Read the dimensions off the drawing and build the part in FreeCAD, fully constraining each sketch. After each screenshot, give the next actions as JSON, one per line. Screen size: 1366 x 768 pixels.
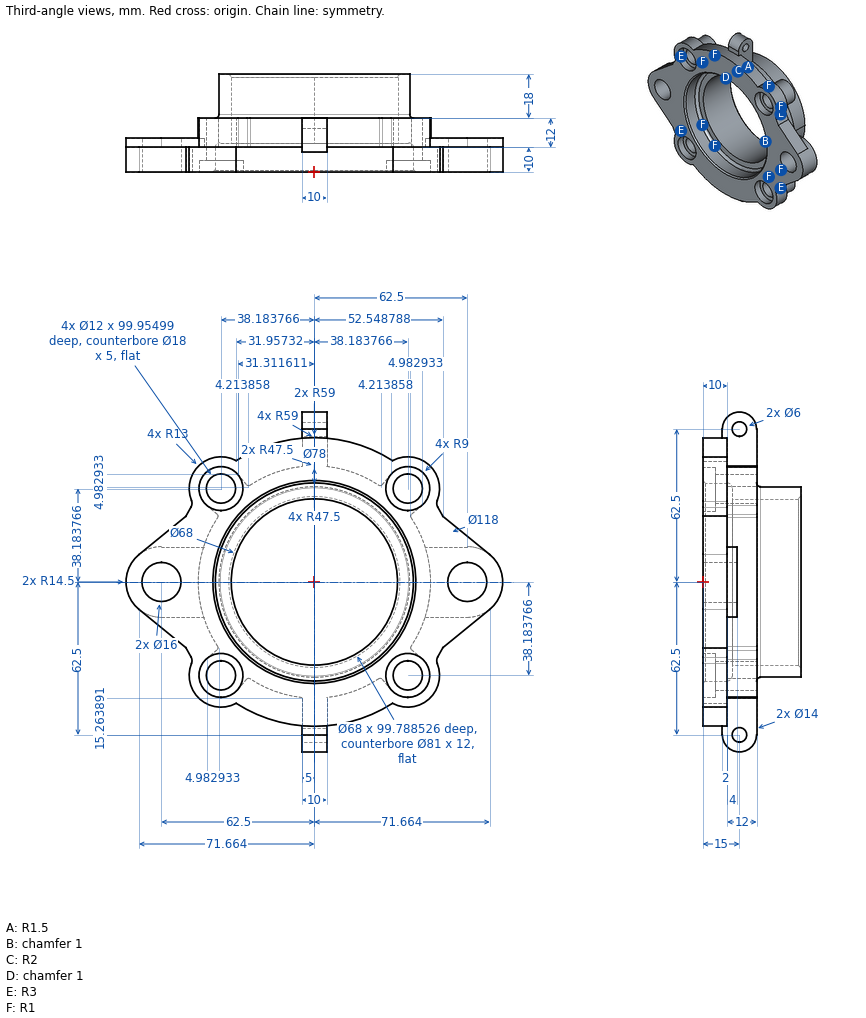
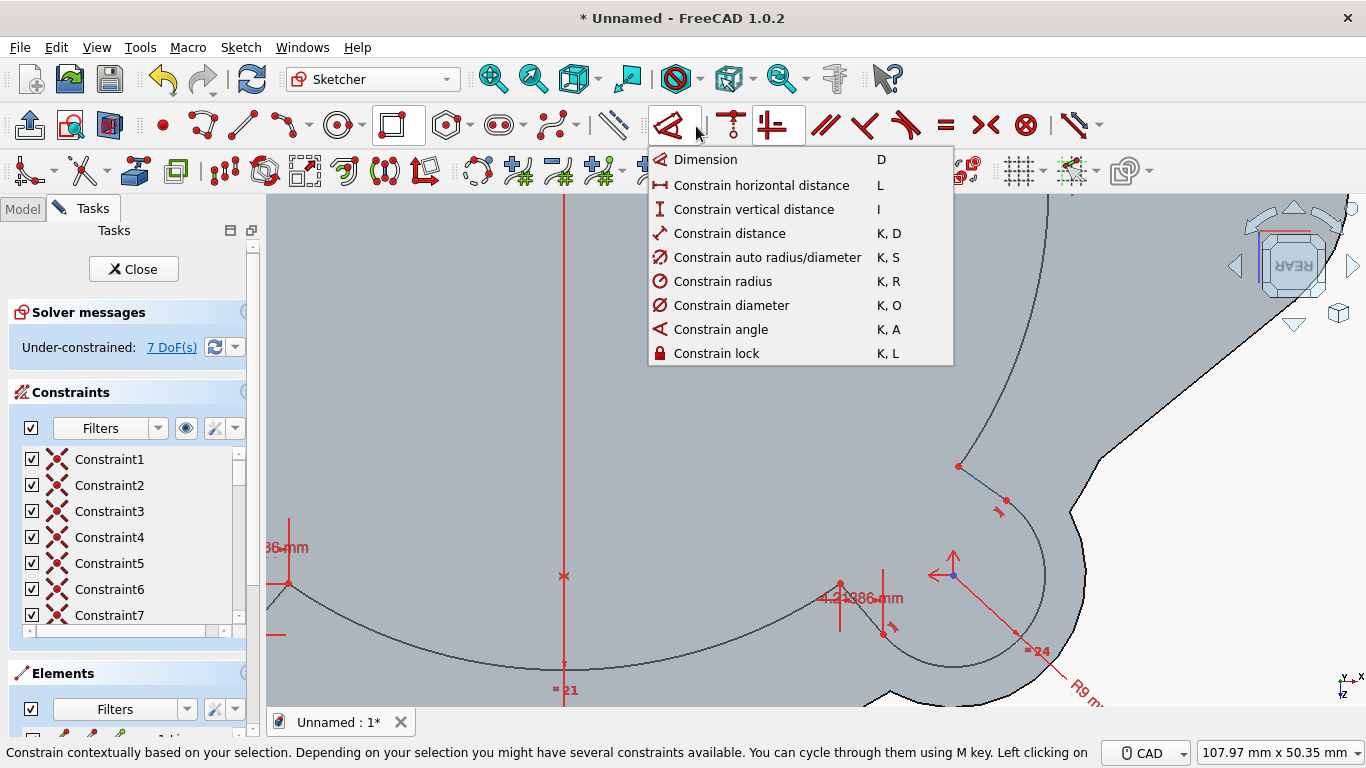
{"action": "left_click", "coordinate": [801, 185]}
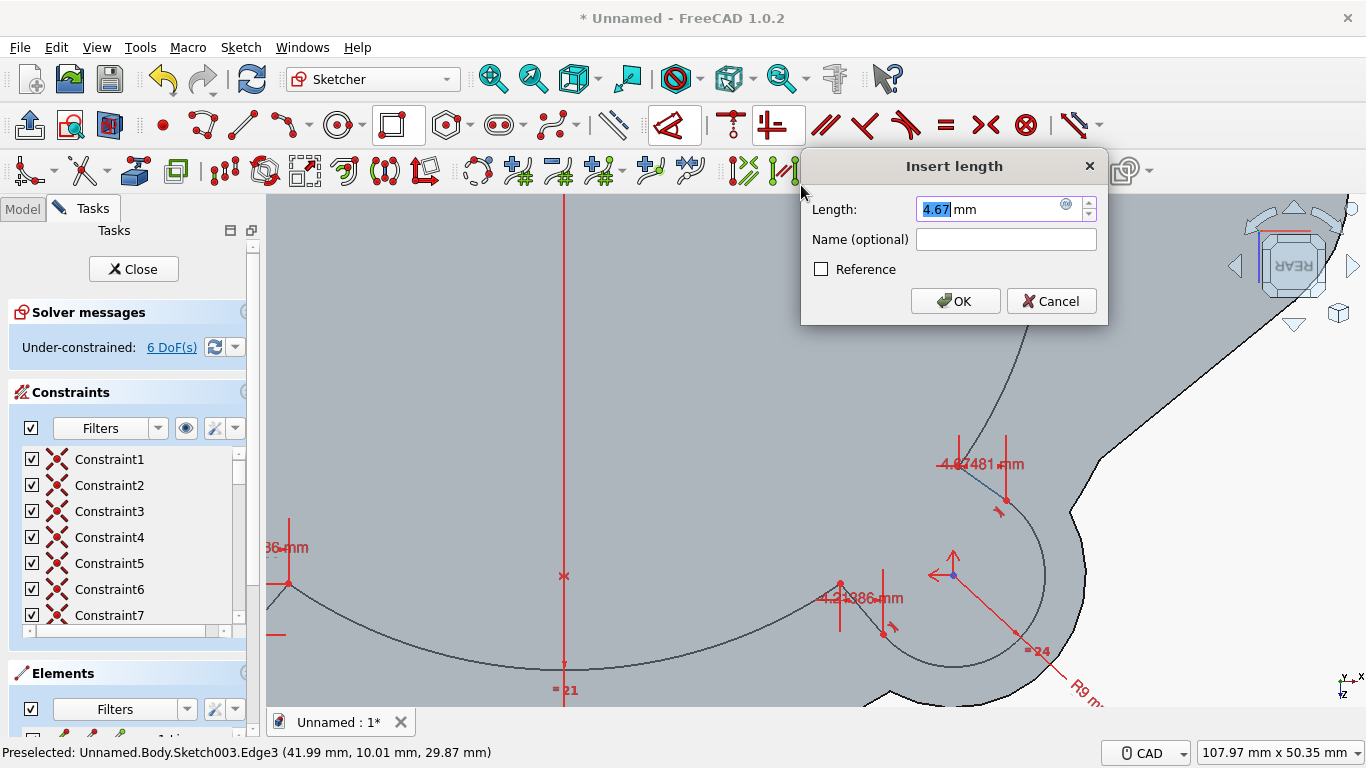
{"action": "type", "text": "4.982933"}
{"action": "key", "text": "Return"}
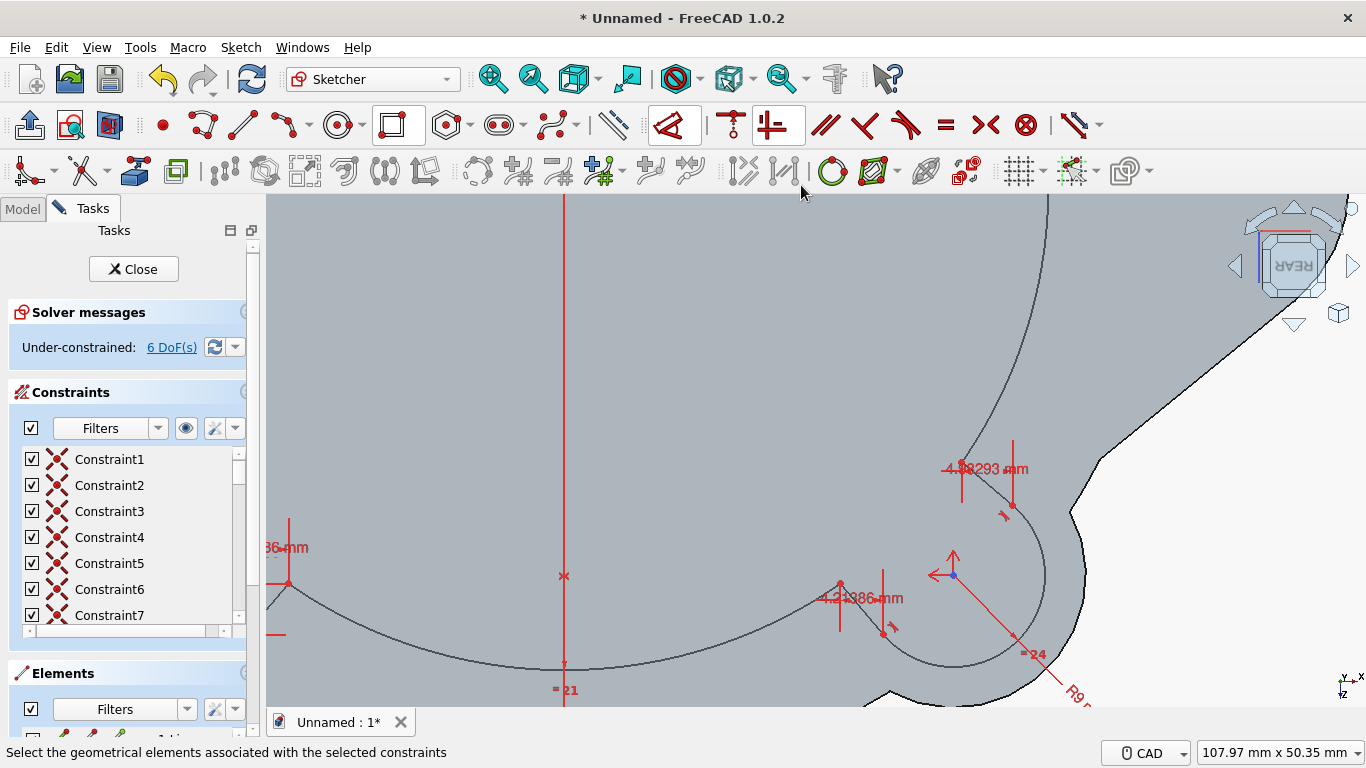
{"action": "scroll", "coordinate": [854, 604], "scroll_direction": "down", "scroll_amount": 5}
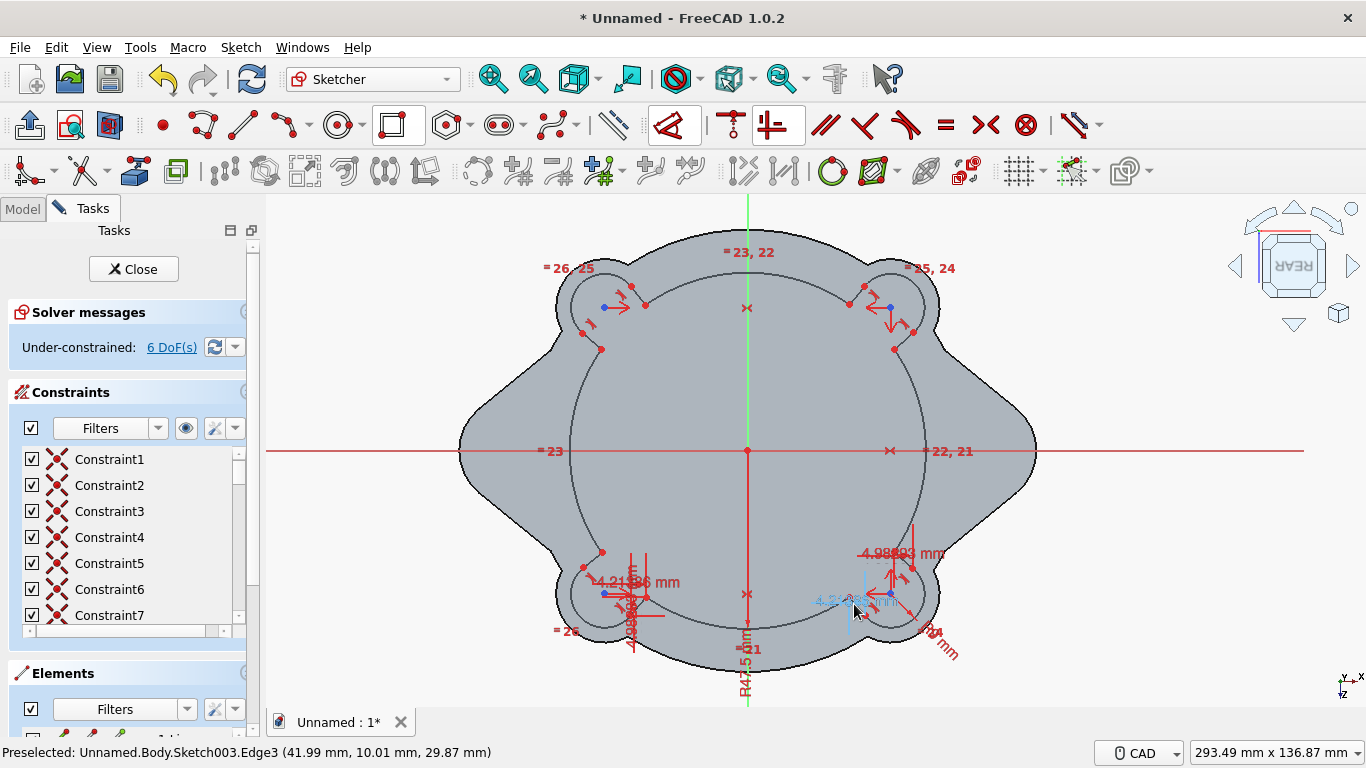
{"action": "scroll", "coordinate": [900, 345], "scroll_direction": "up", "scroll_amount": 4}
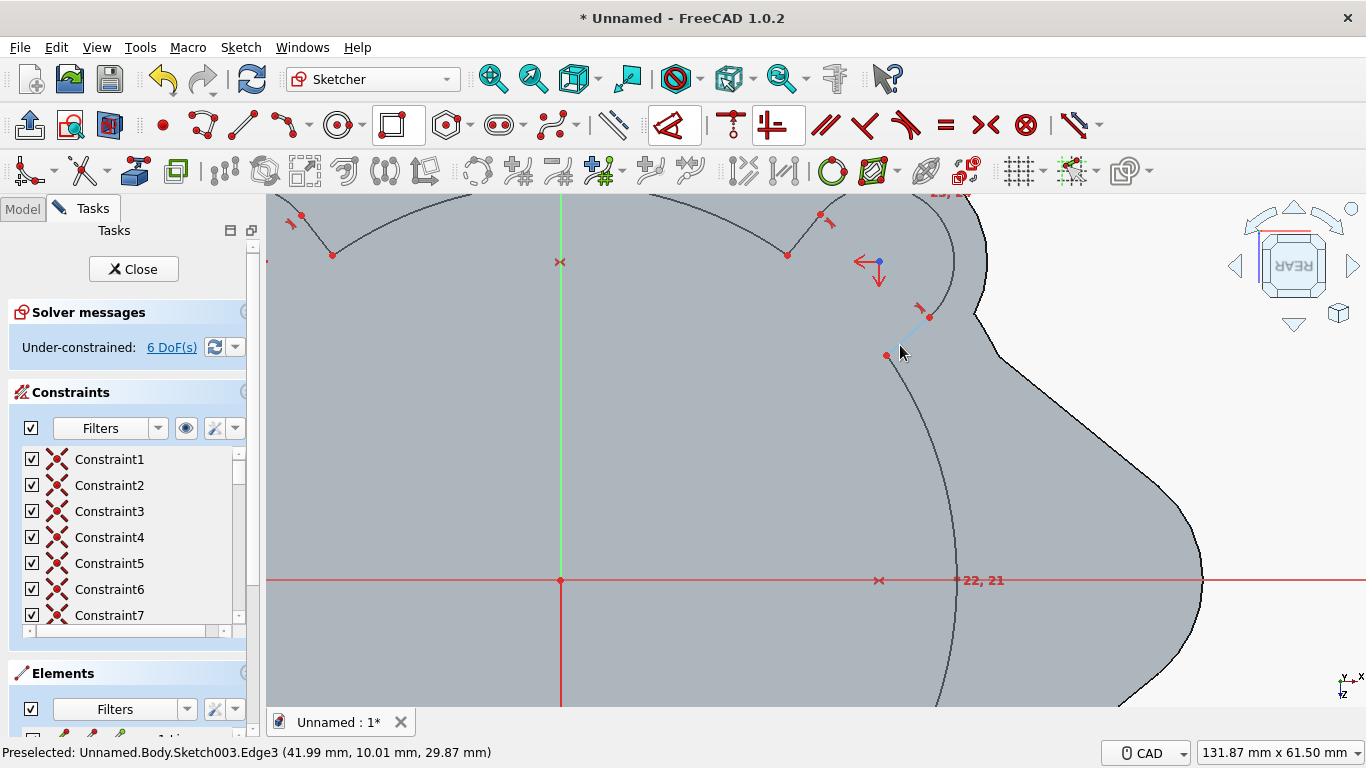
{"action": "left_click", "coordinate": [900, 344]}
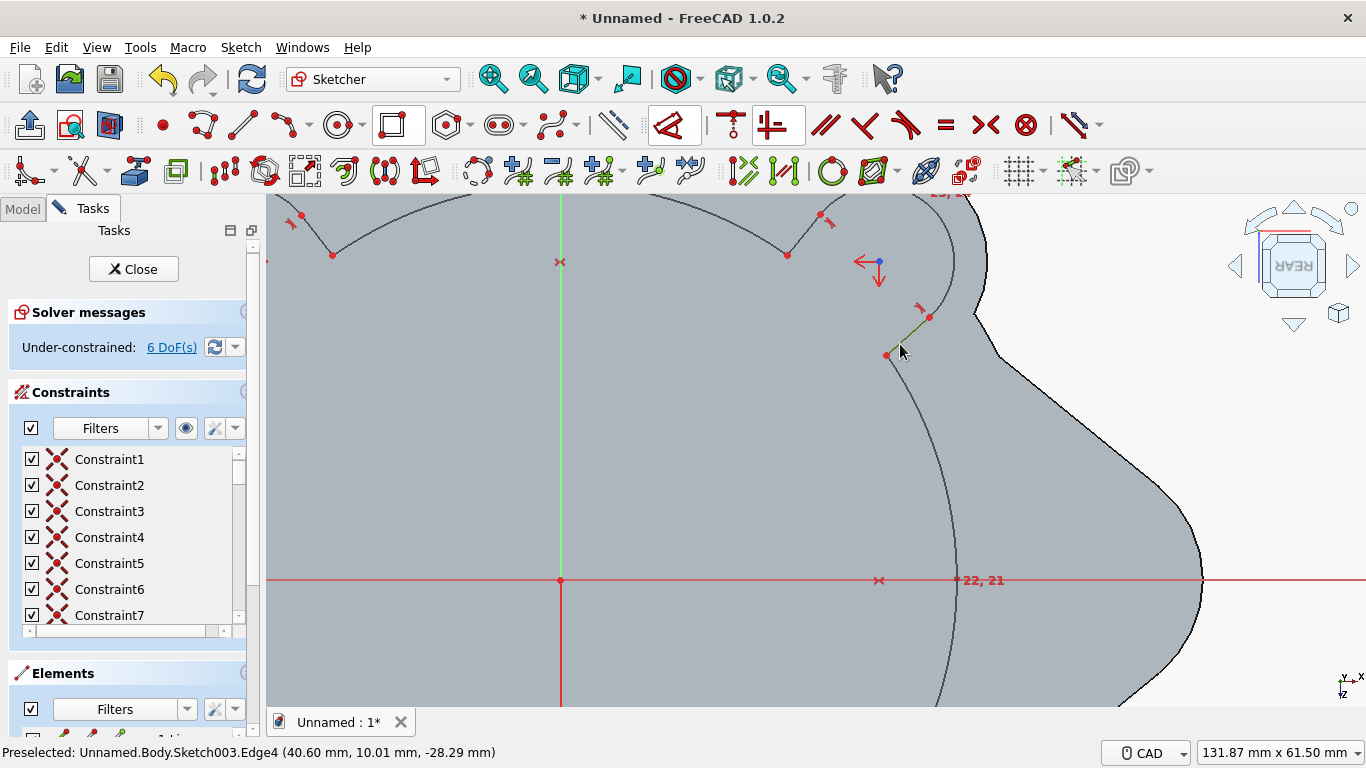
{"action": "left_click", "coordinate": [696, 126]}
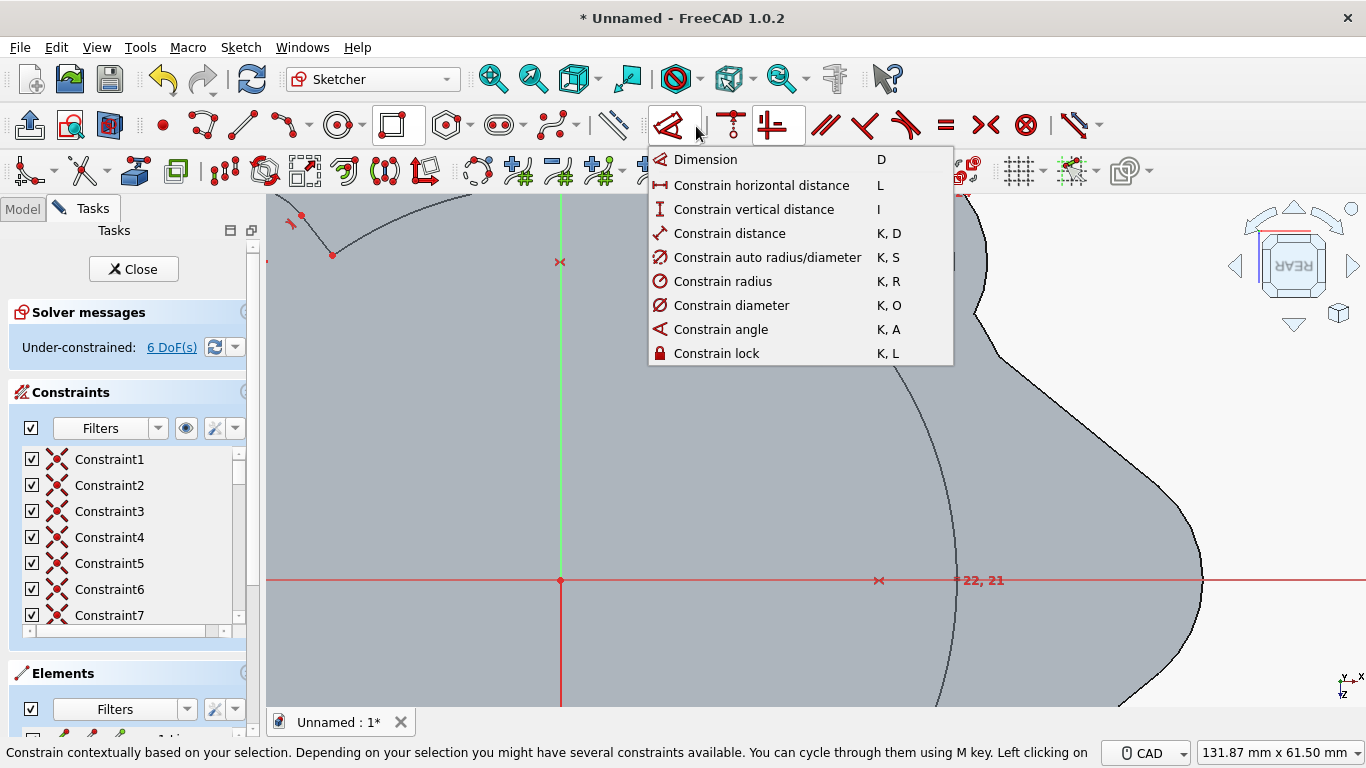
{"action": "left_click", "coordinate": [801, 185]}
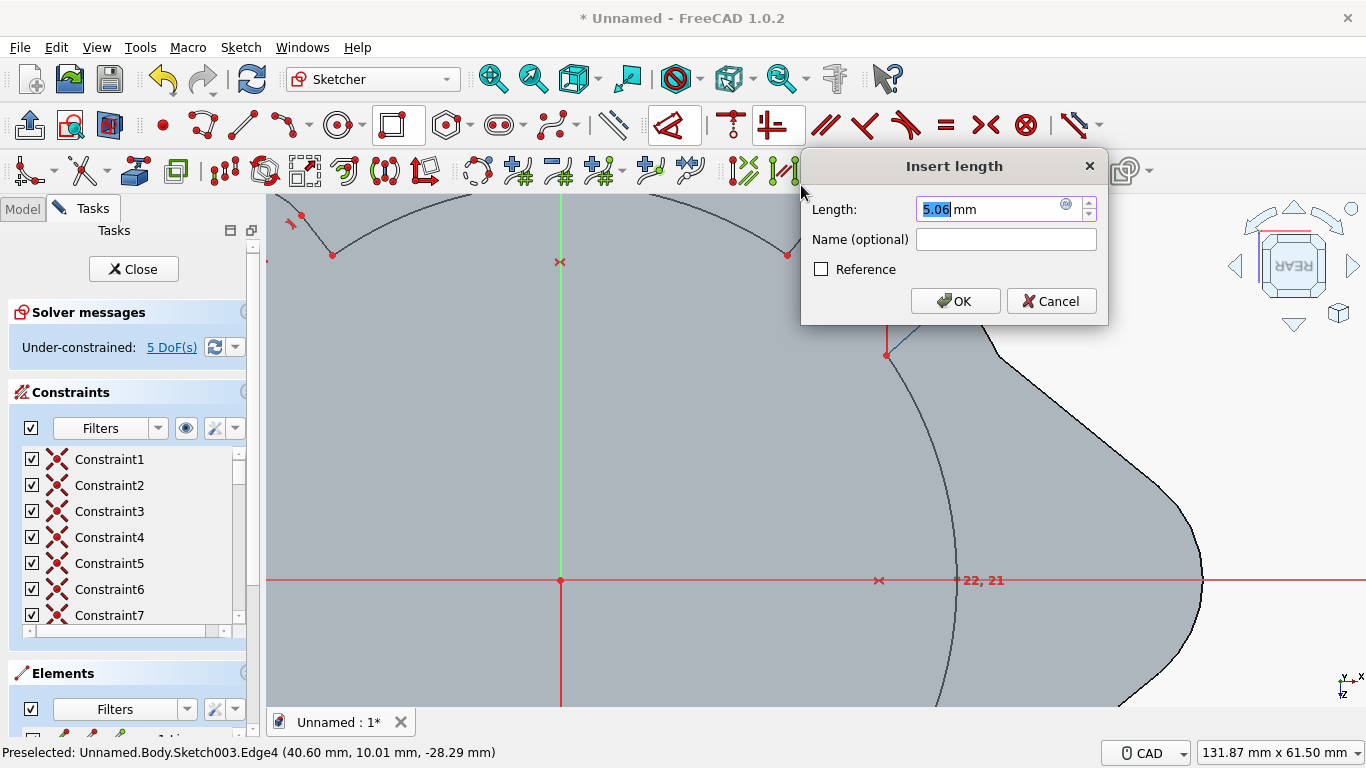
{"action": "type", "text": "4.982933"}
{"action": "key", "text": "Return"}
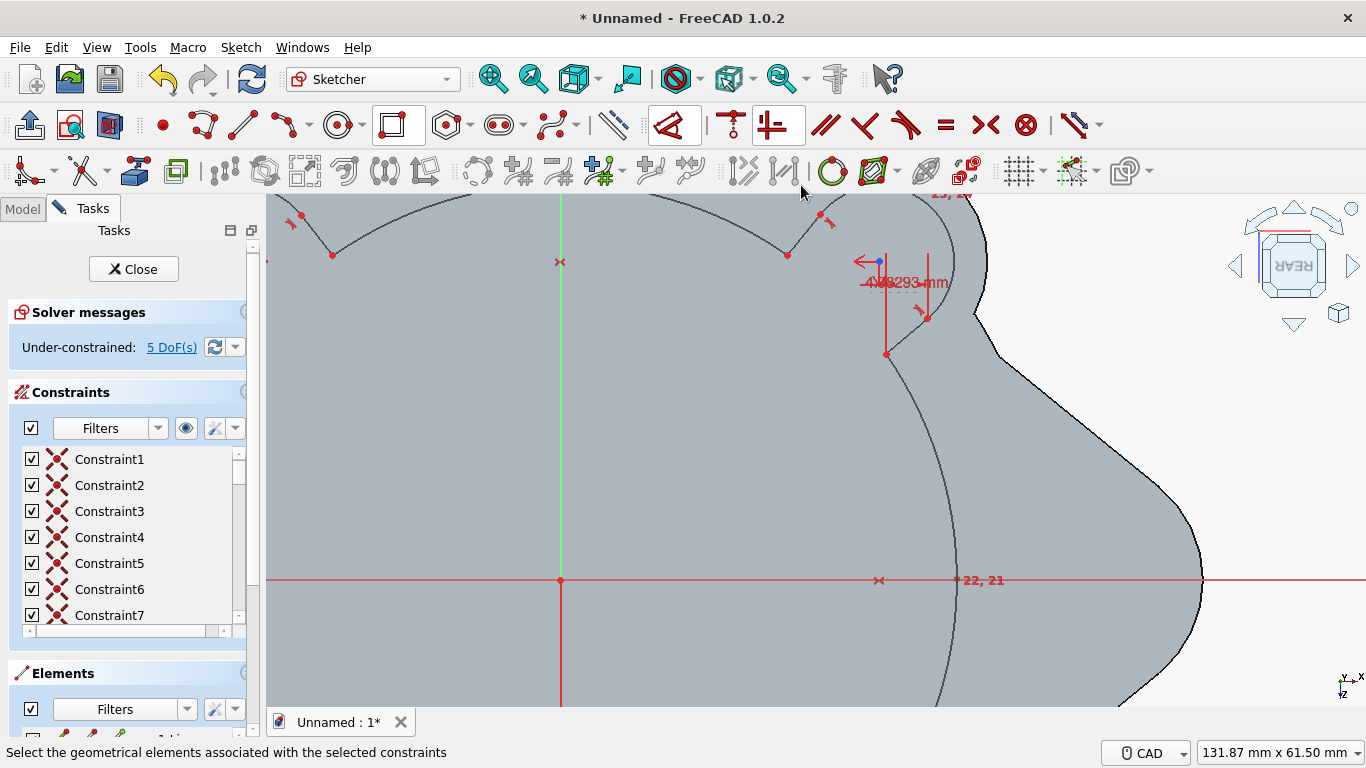
{"action": "left_click", "coordinate": [811, 227]}